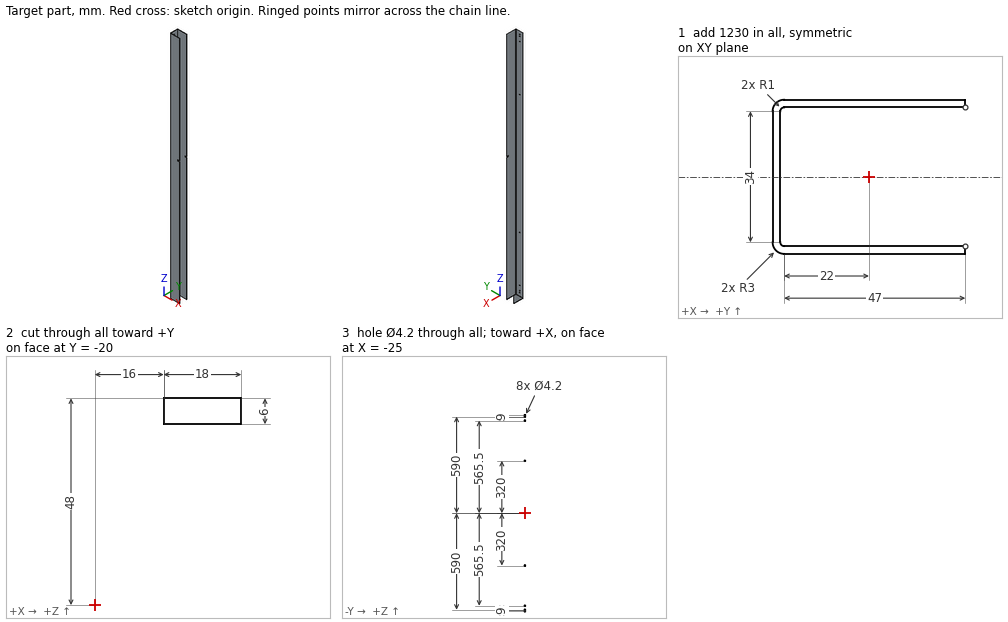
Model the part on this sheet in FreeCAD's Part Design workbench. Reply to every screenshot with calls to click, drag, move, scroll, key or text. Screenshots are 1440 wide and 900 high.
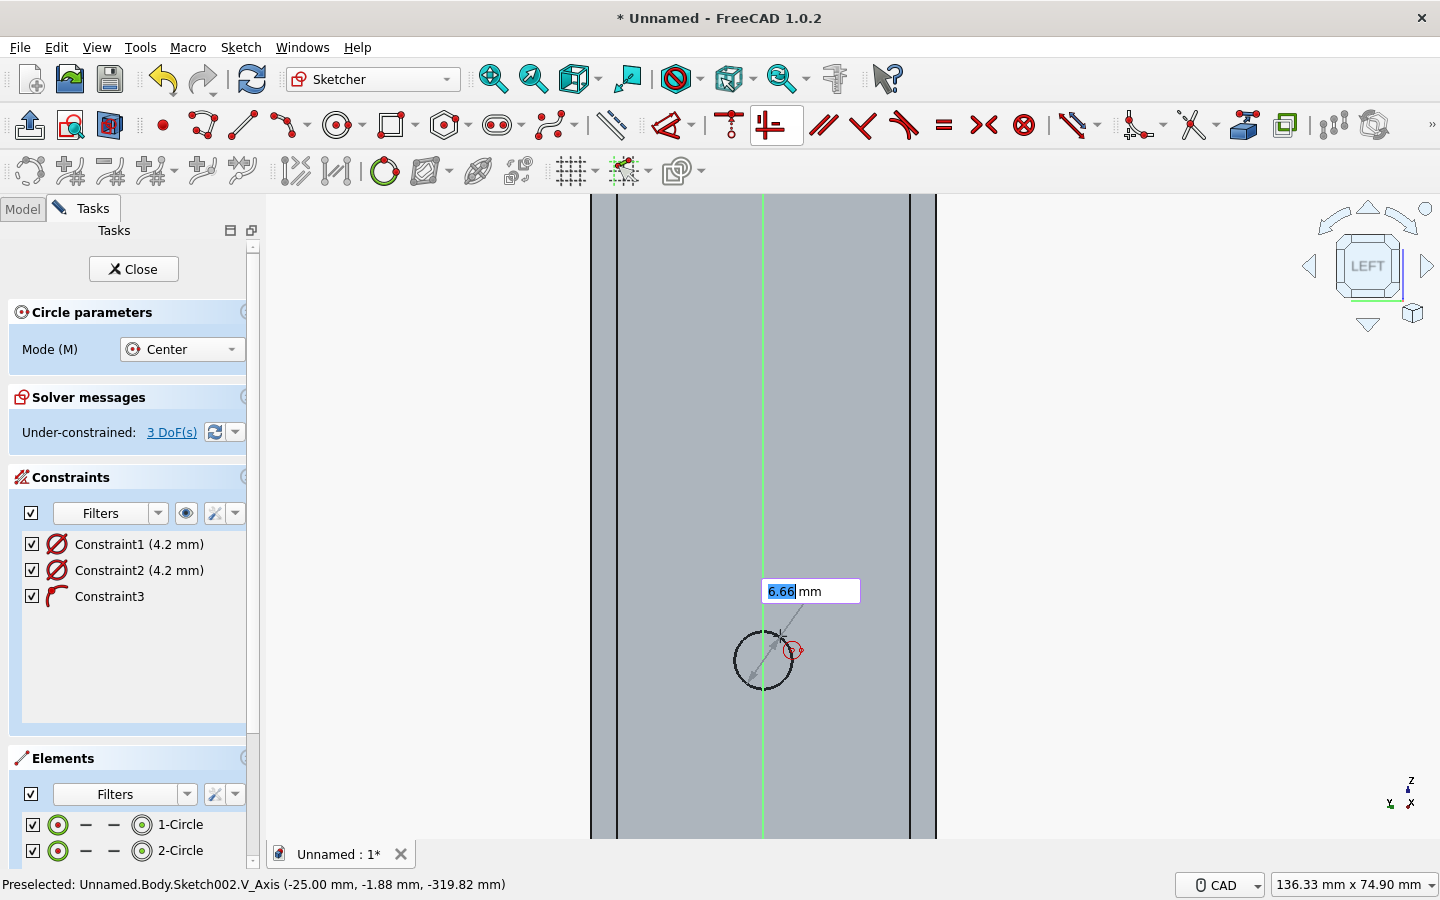
text(4.2)
key(Return)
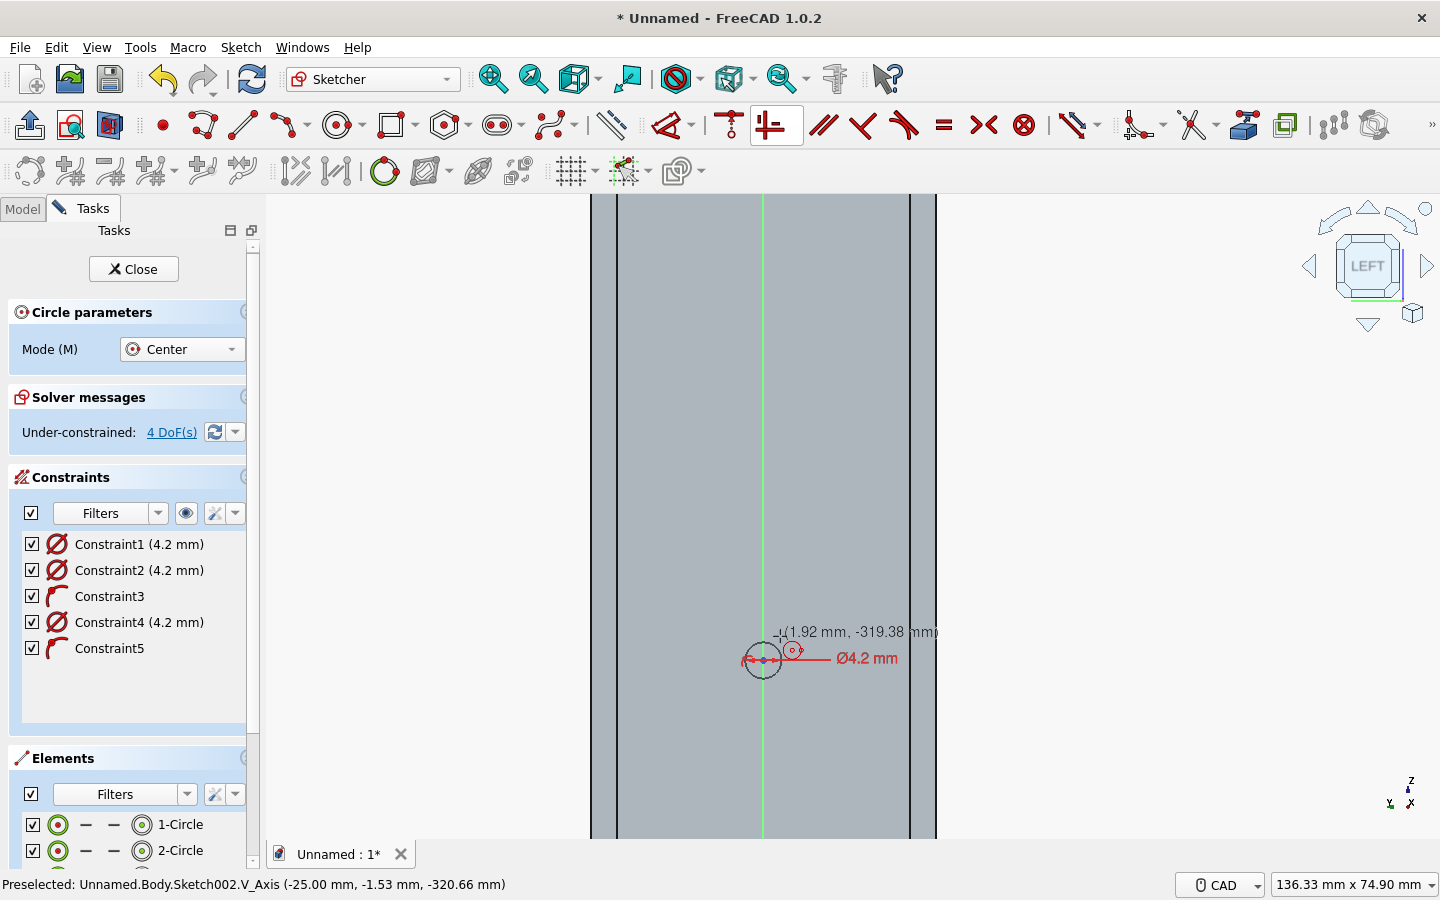
scroll(786, 654, down, 15)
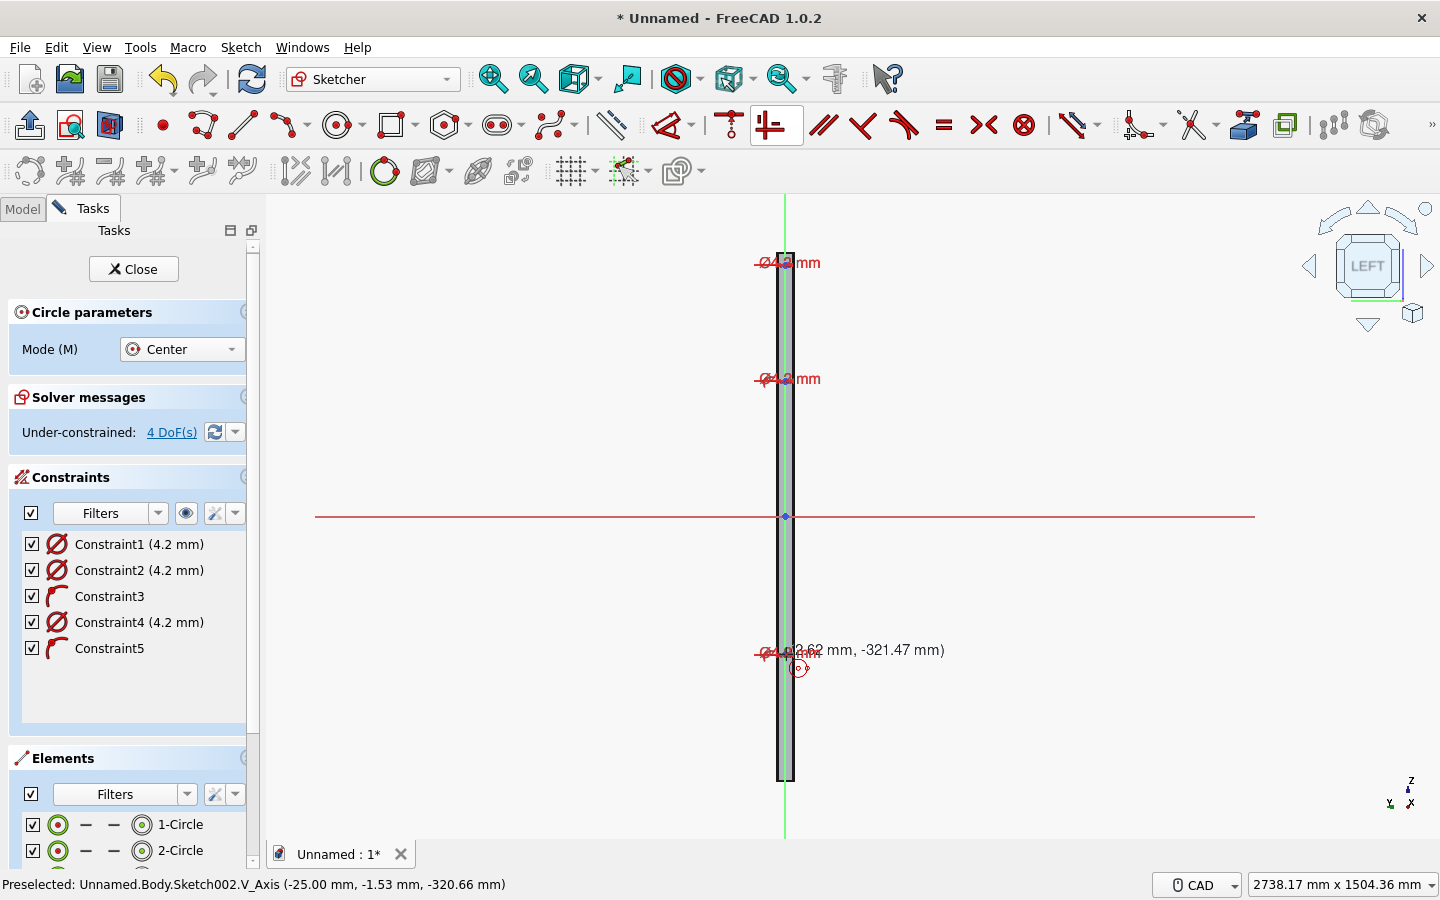
scroll(785, 770, up, 17)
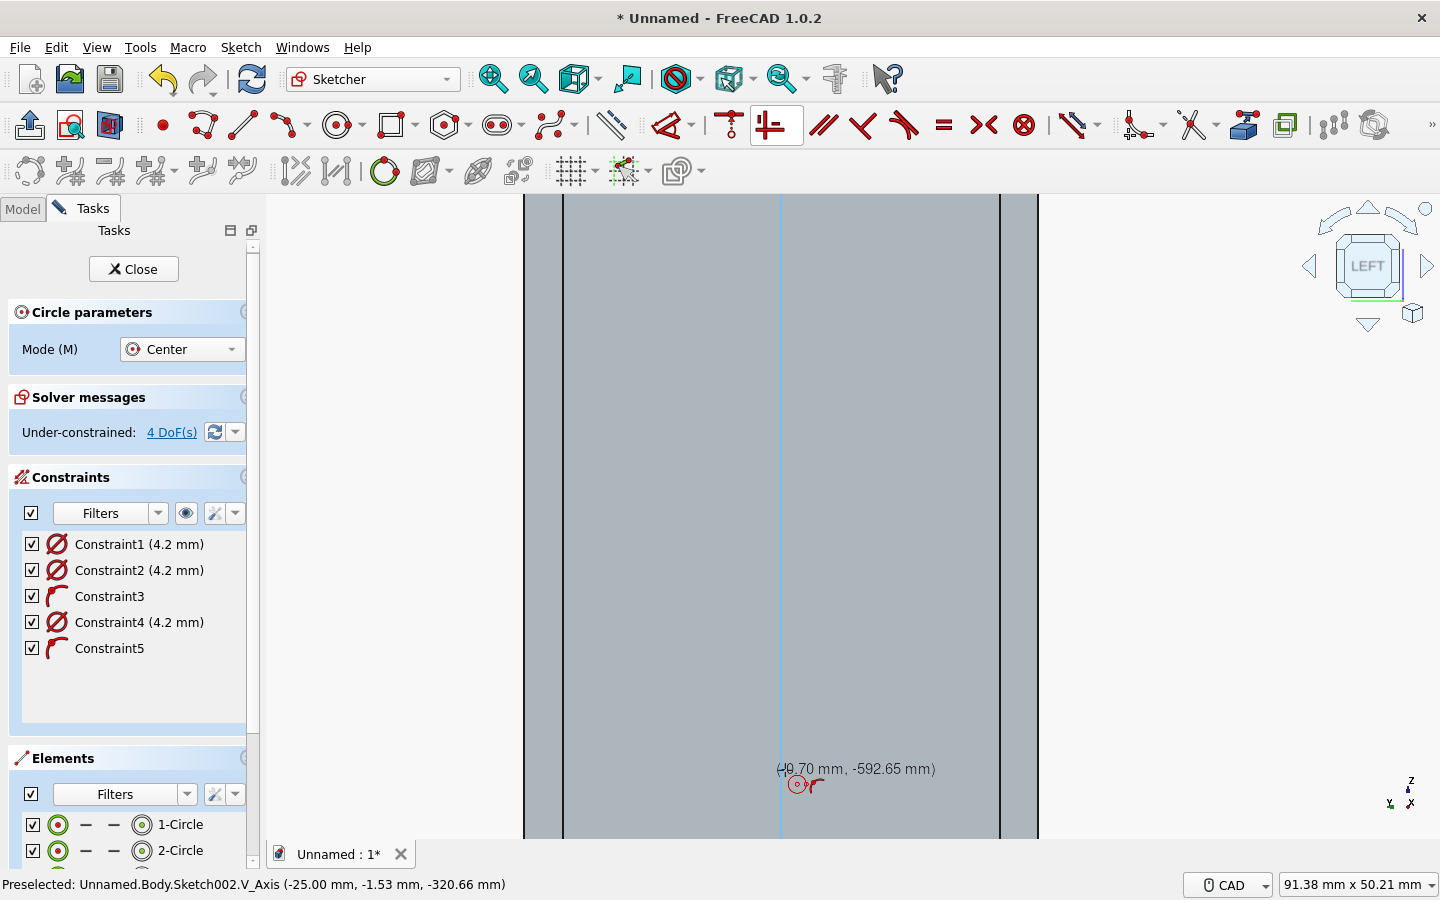
scroll(785, 770, down, 17)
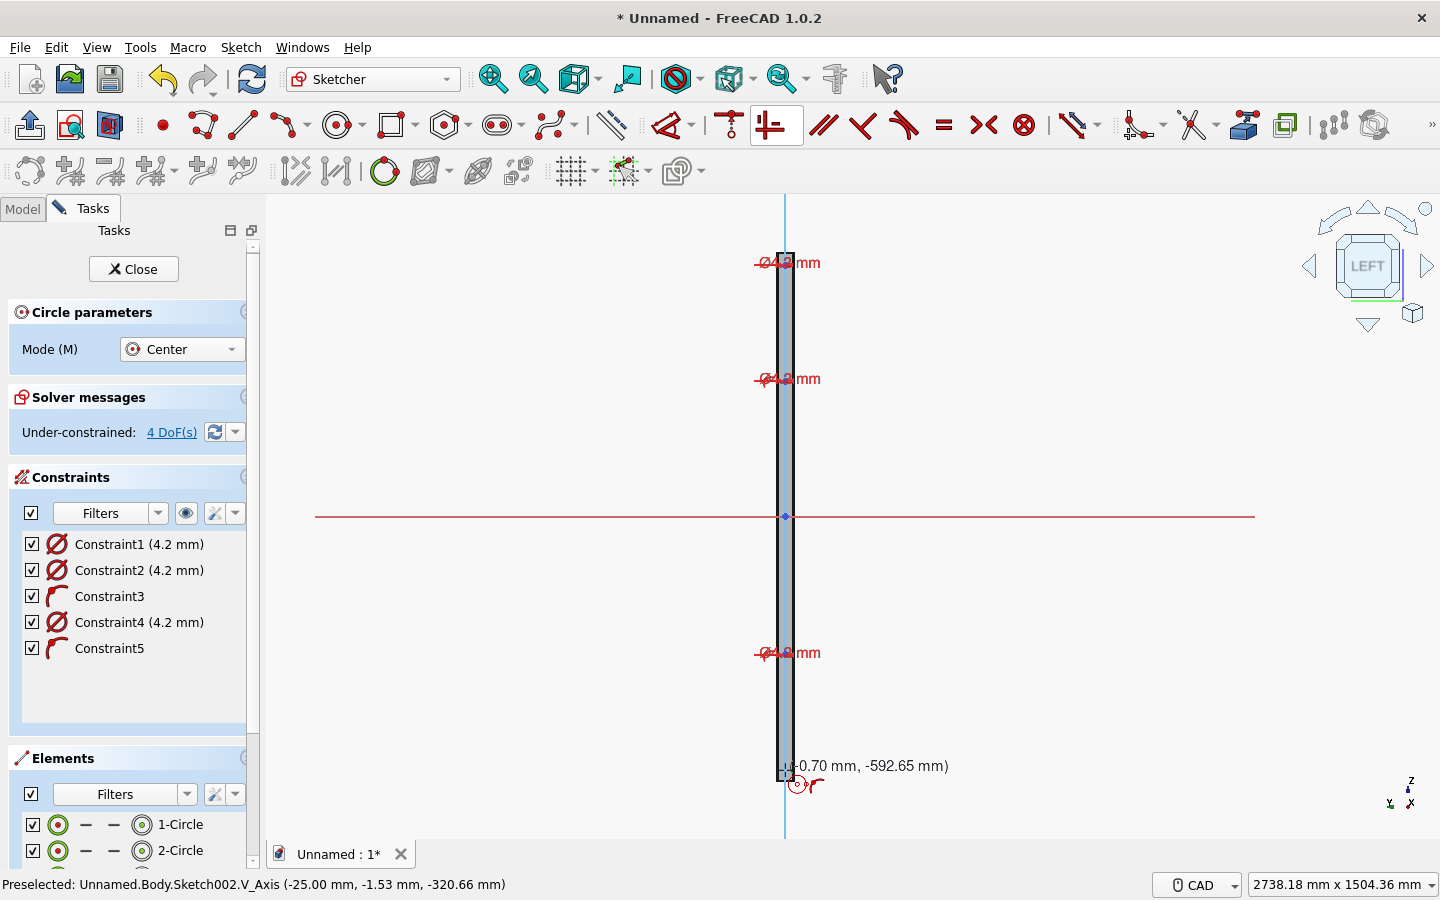
click(785, 770)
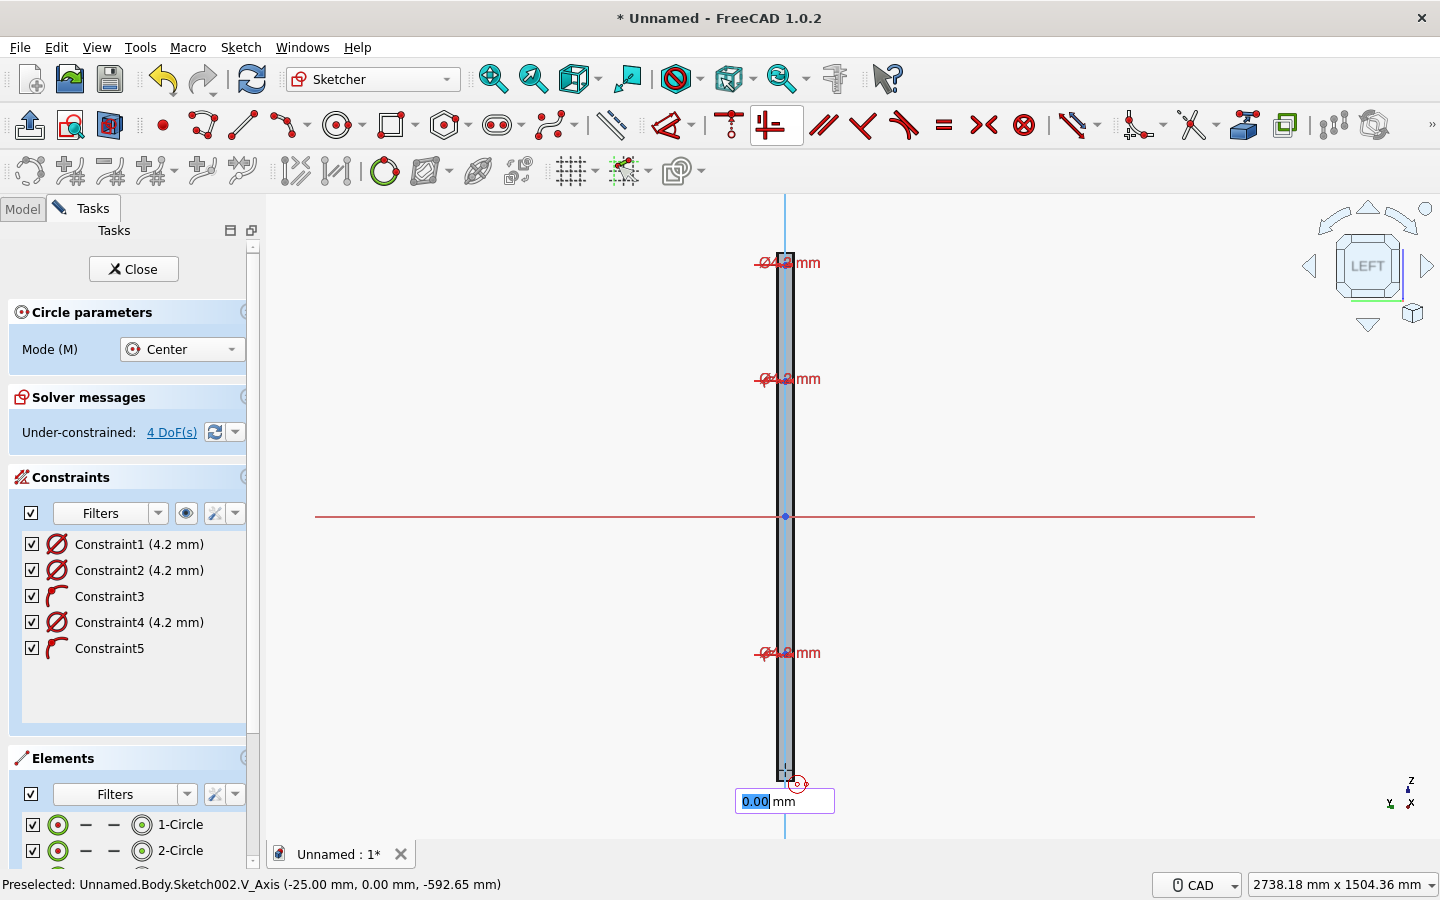
scroll(786, 770, up, 15)
move(780, 744)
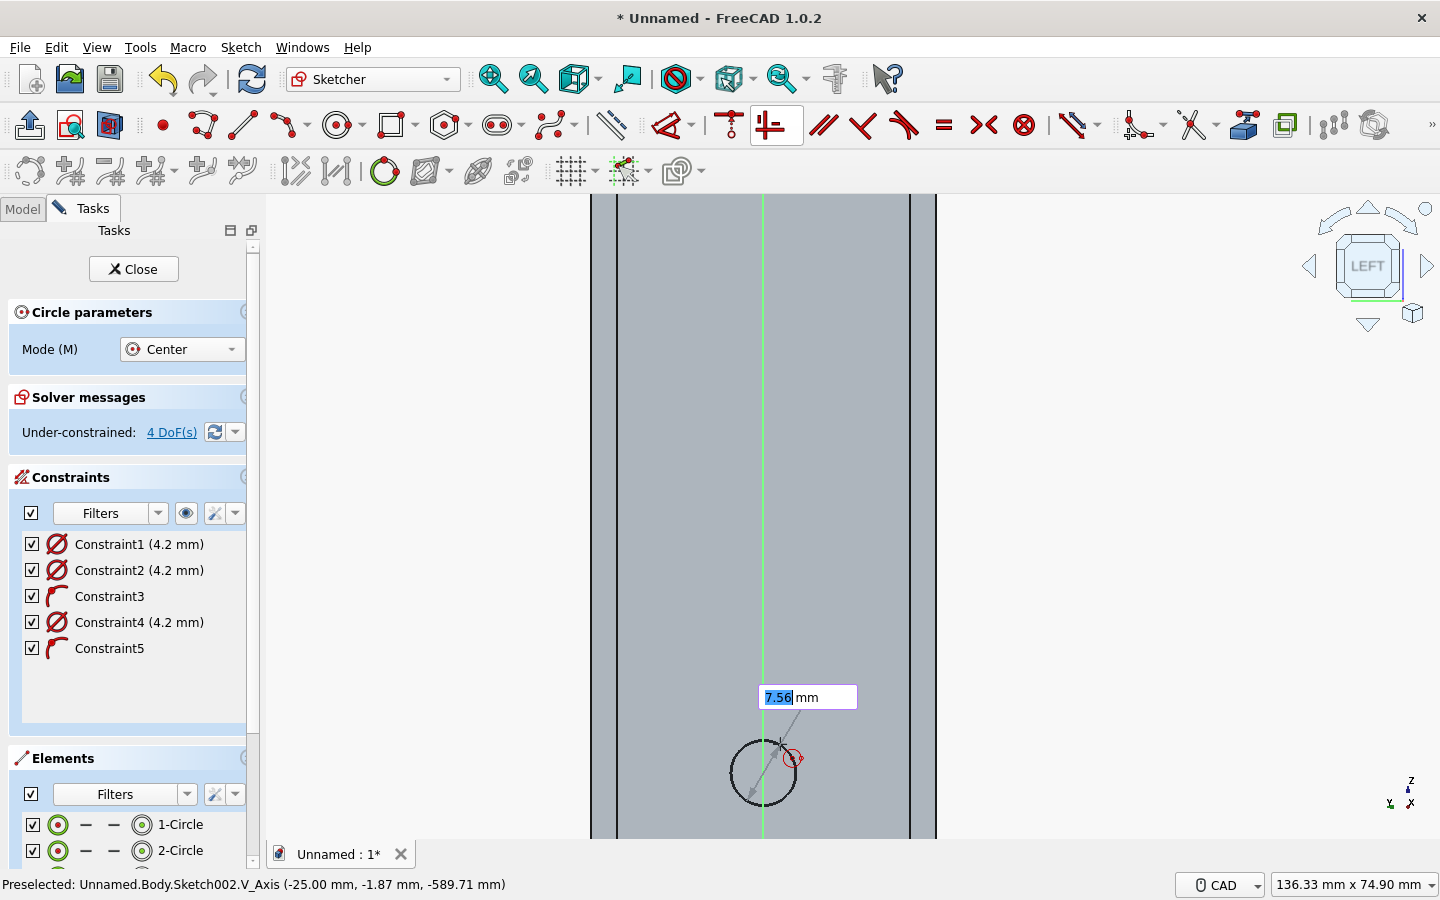
text(4.2)
key(Return)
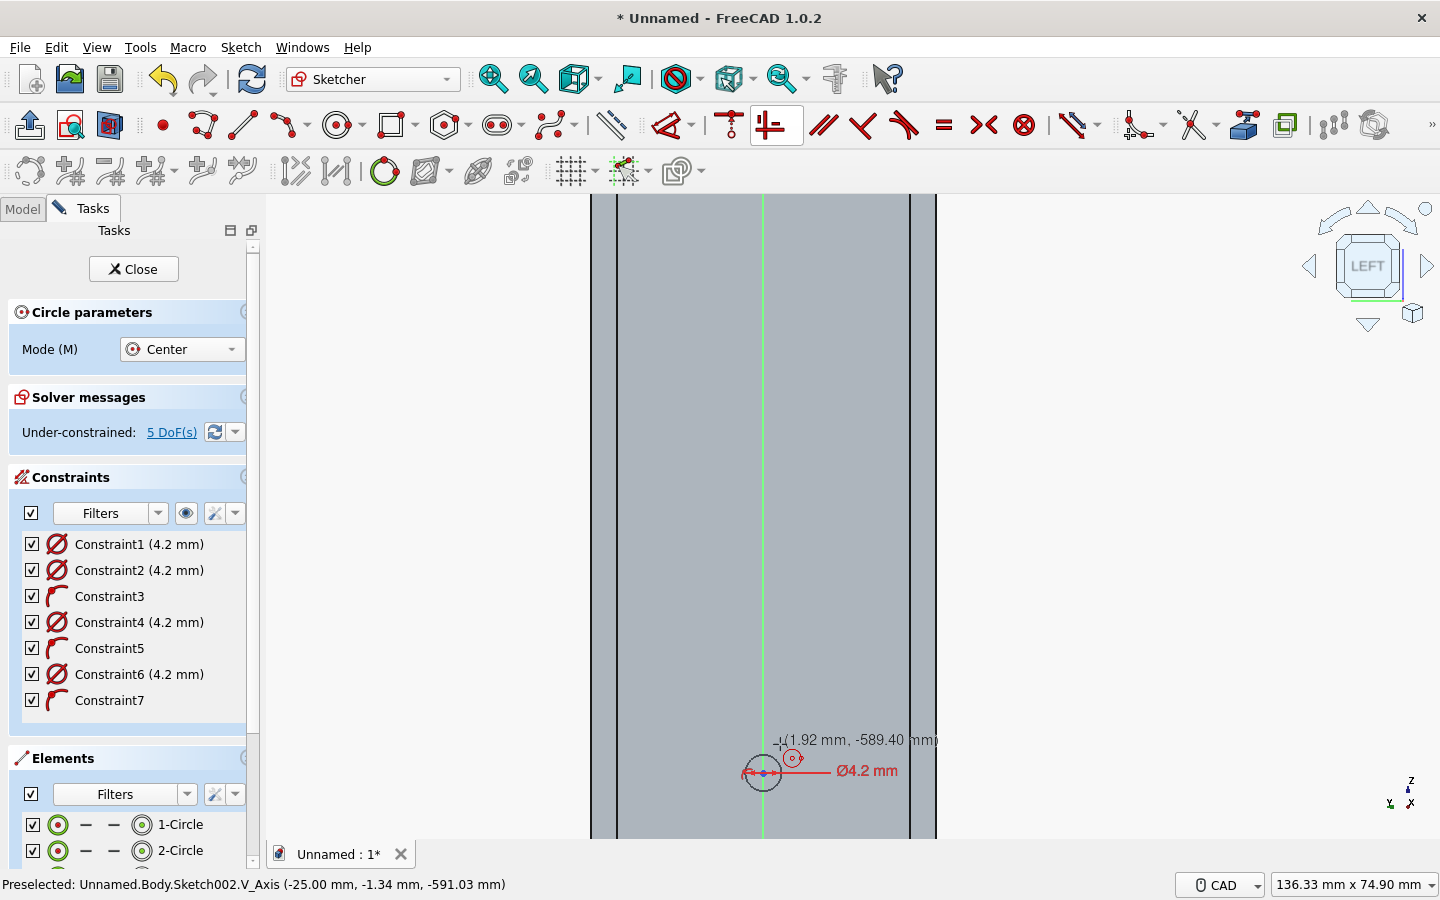
scroll(786, 770, down, 15)